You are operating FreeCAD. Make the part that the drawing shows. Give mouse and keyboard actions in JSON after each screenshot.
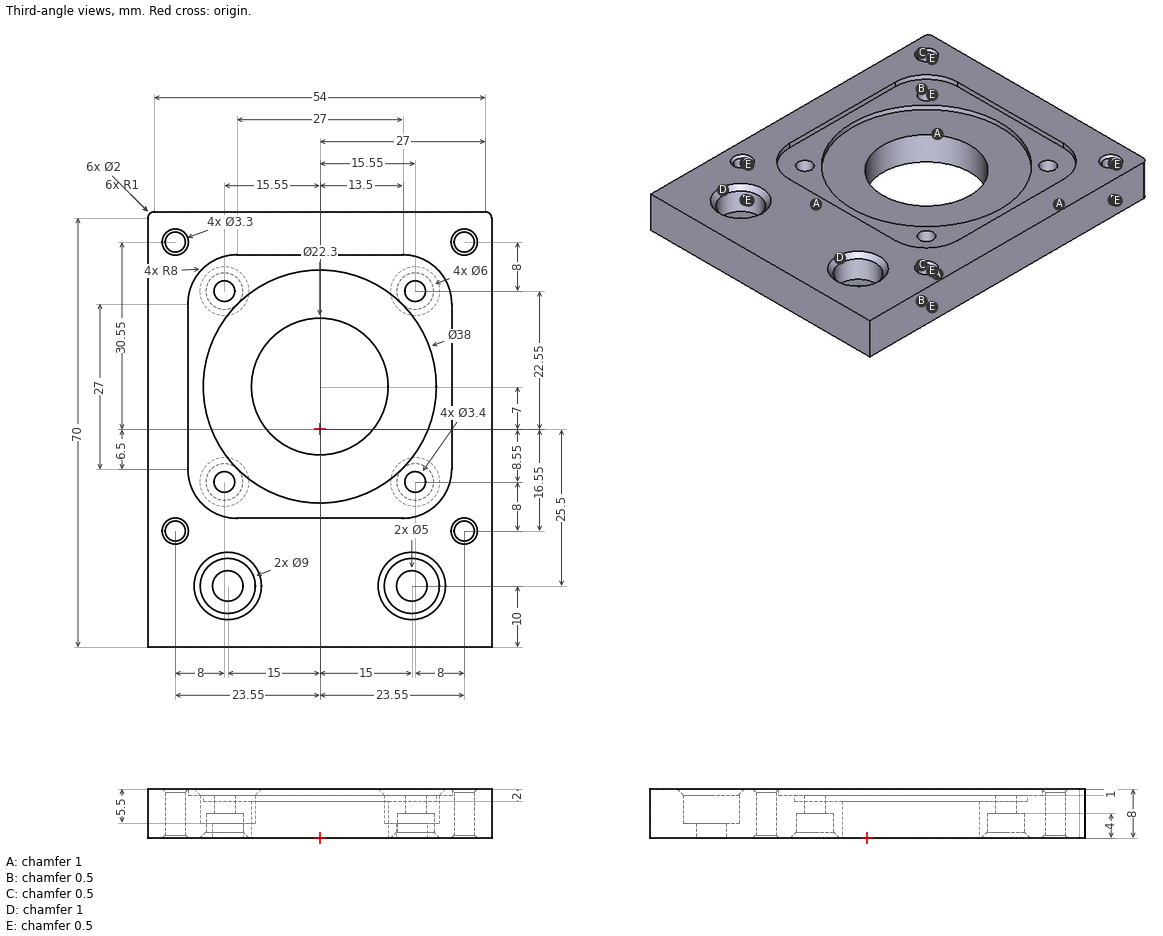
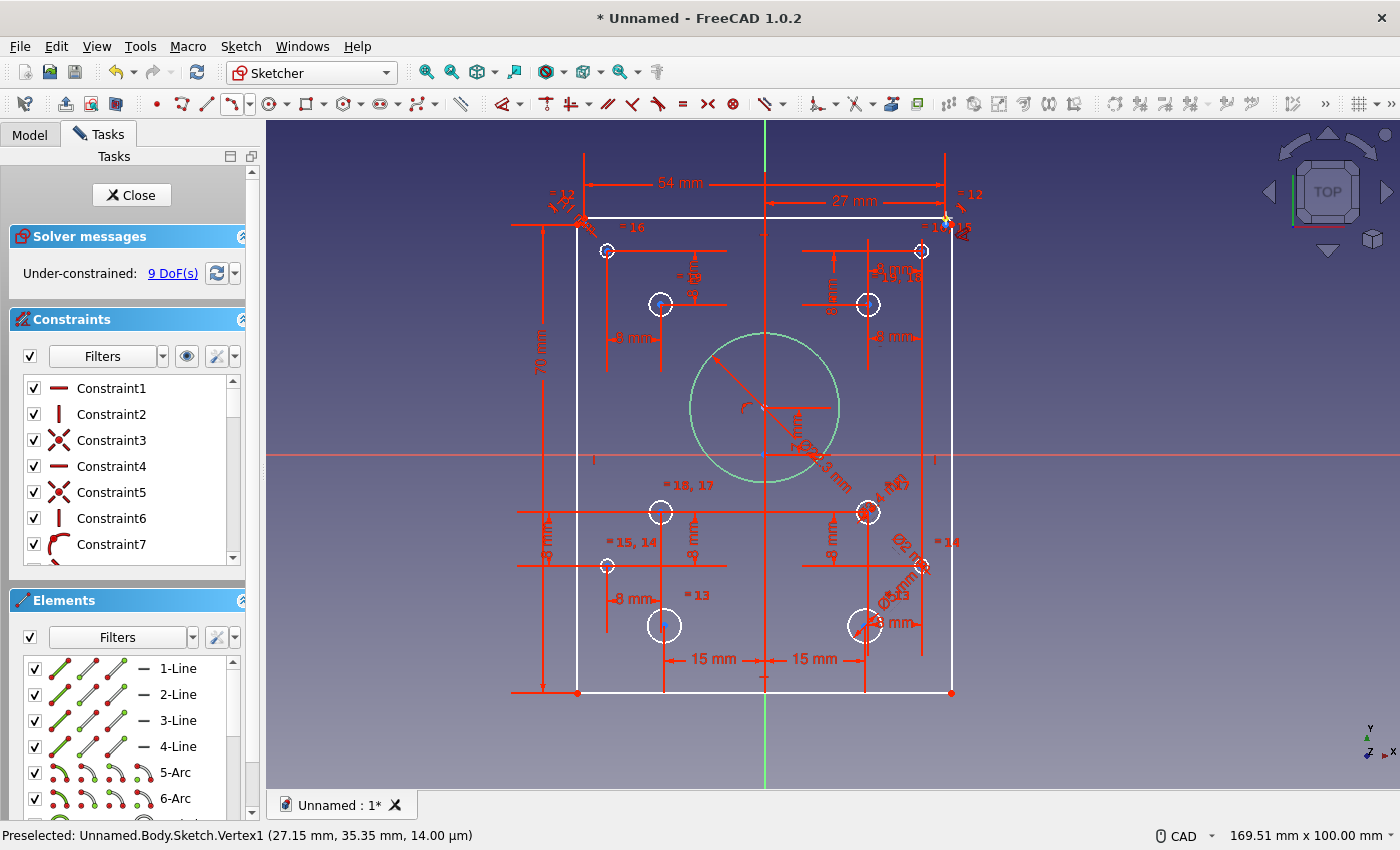
{"action": "left_click", "coordinate": [952, 693]}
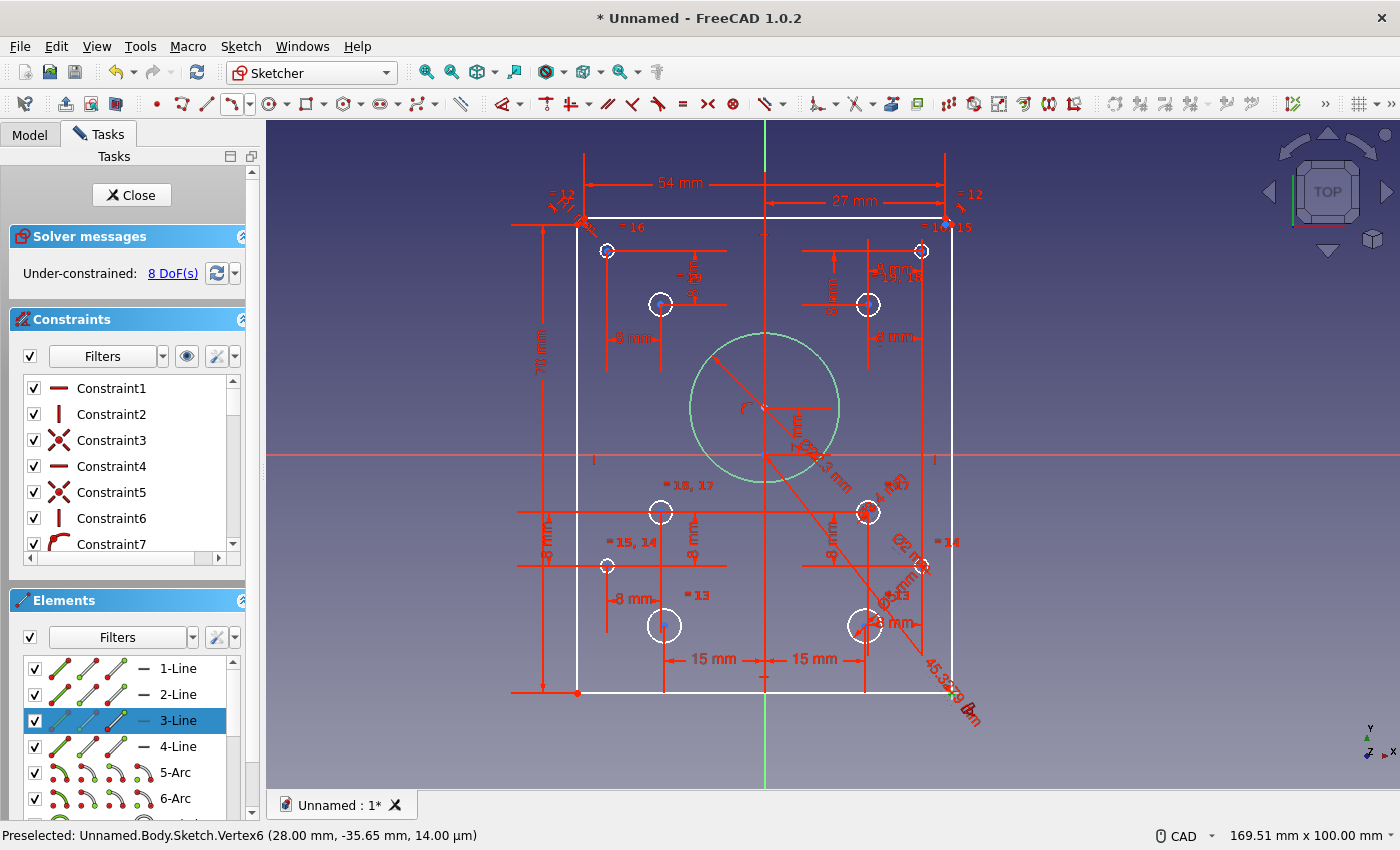
{"action": "left_click", "coordinate": [865, 626]}
{"action": "left_click", "coordinate": [986, 660]}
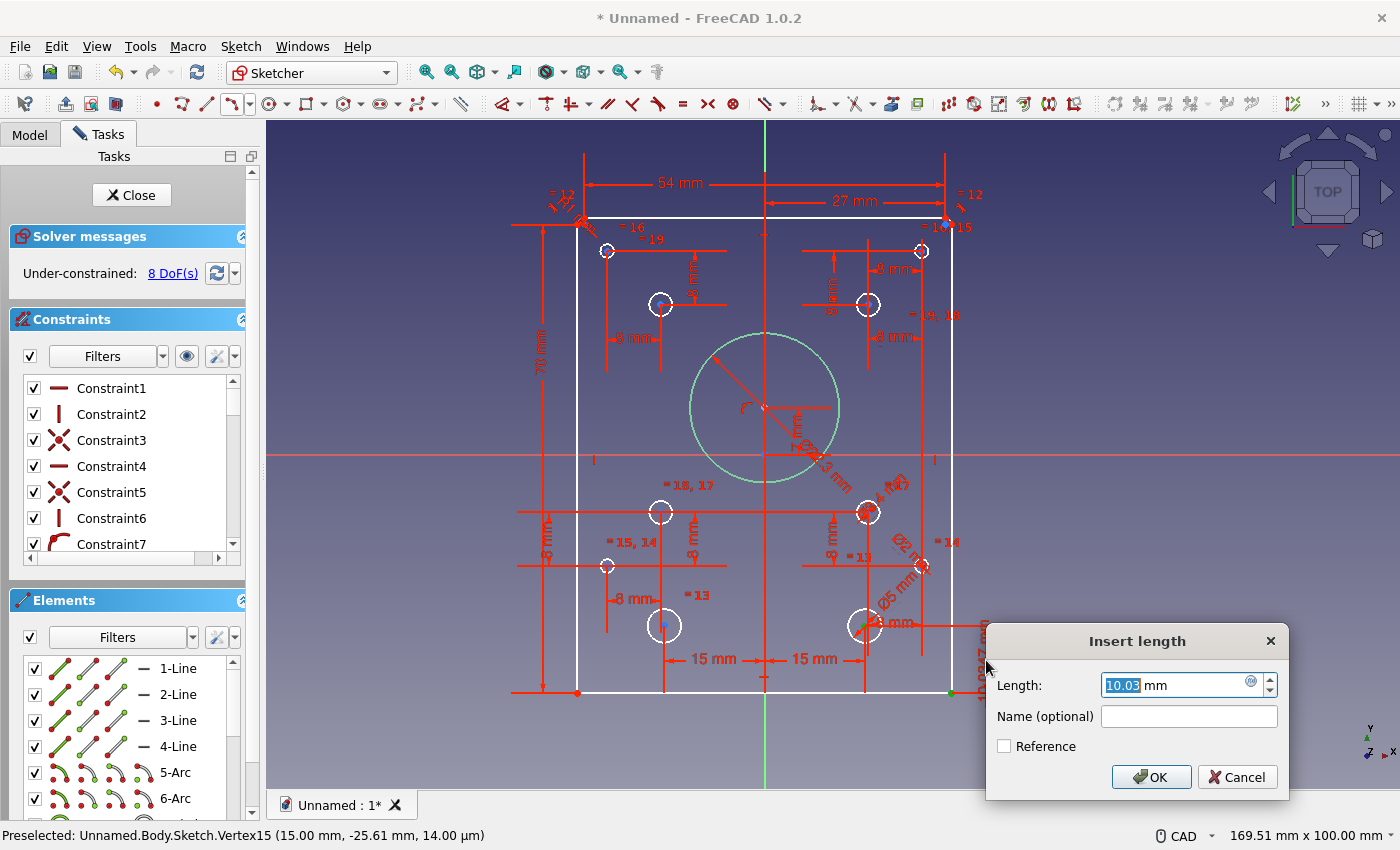
{"action": "type", "text": "10"}
{"action": "key", "text": "Return"}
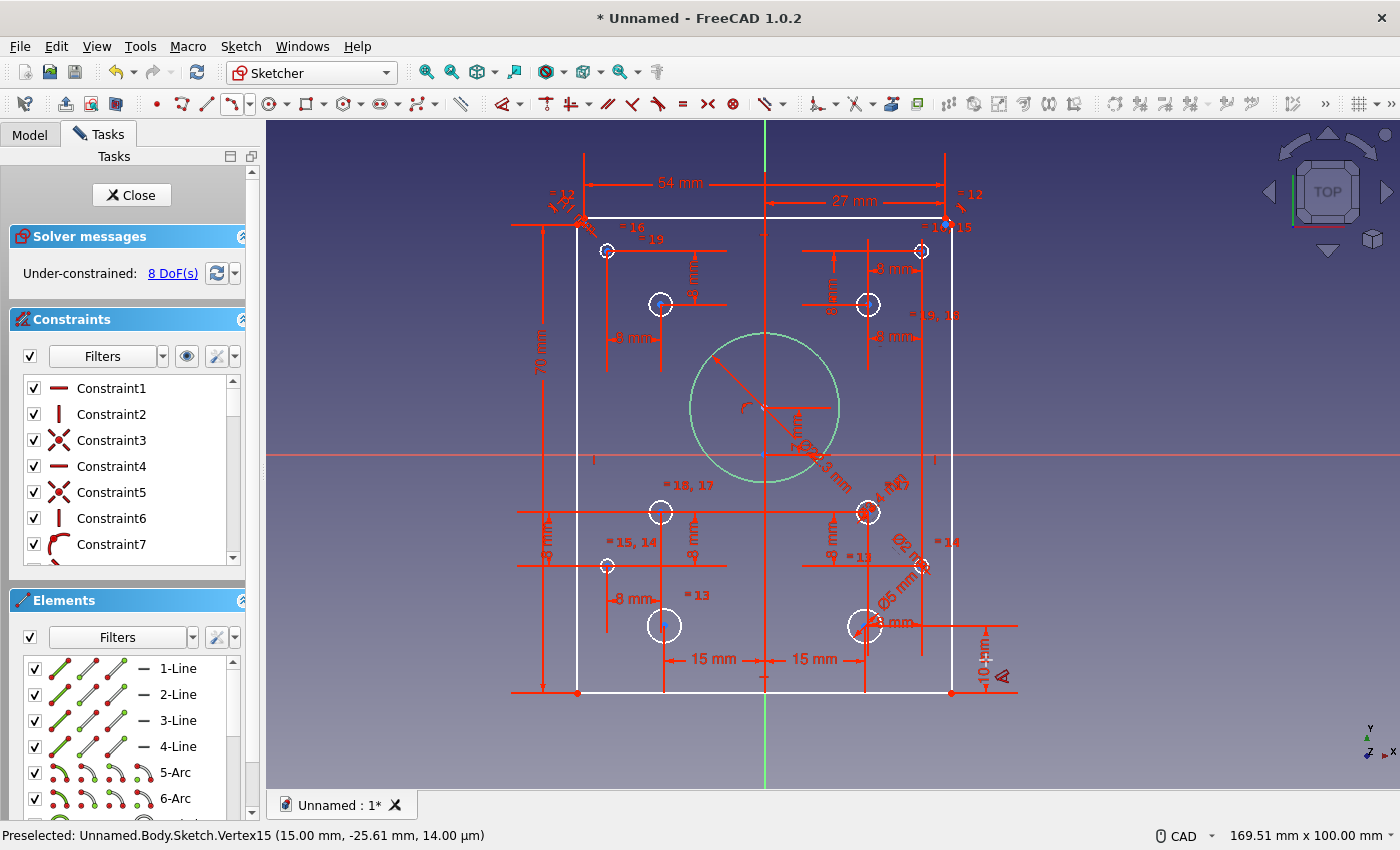
{"action": "left_click", "coordinate": [577, 693]}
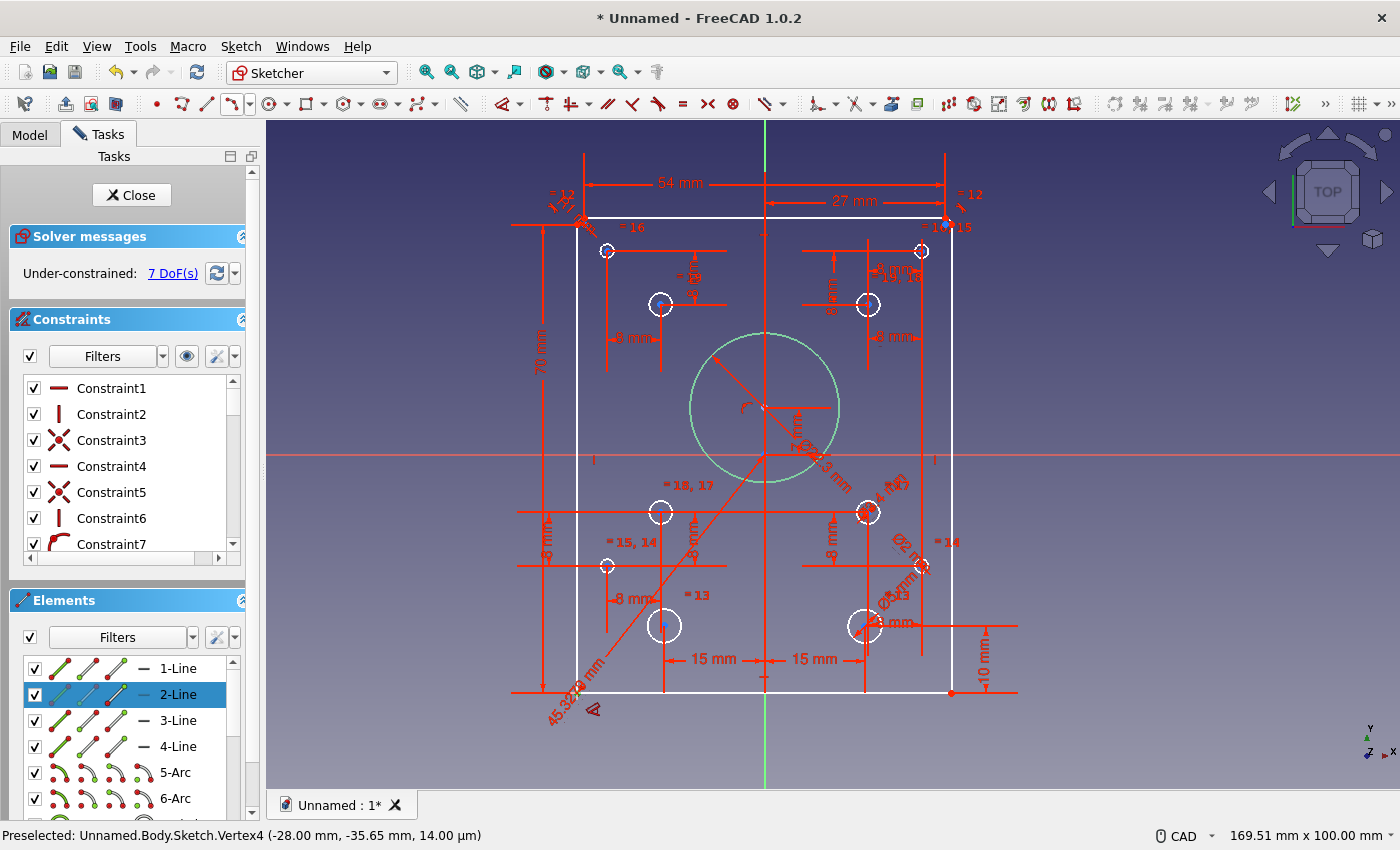
{"action": "left_click", "coordinate": [664, 626]}
{"action": "left_click", "coordinate": [543, 660]}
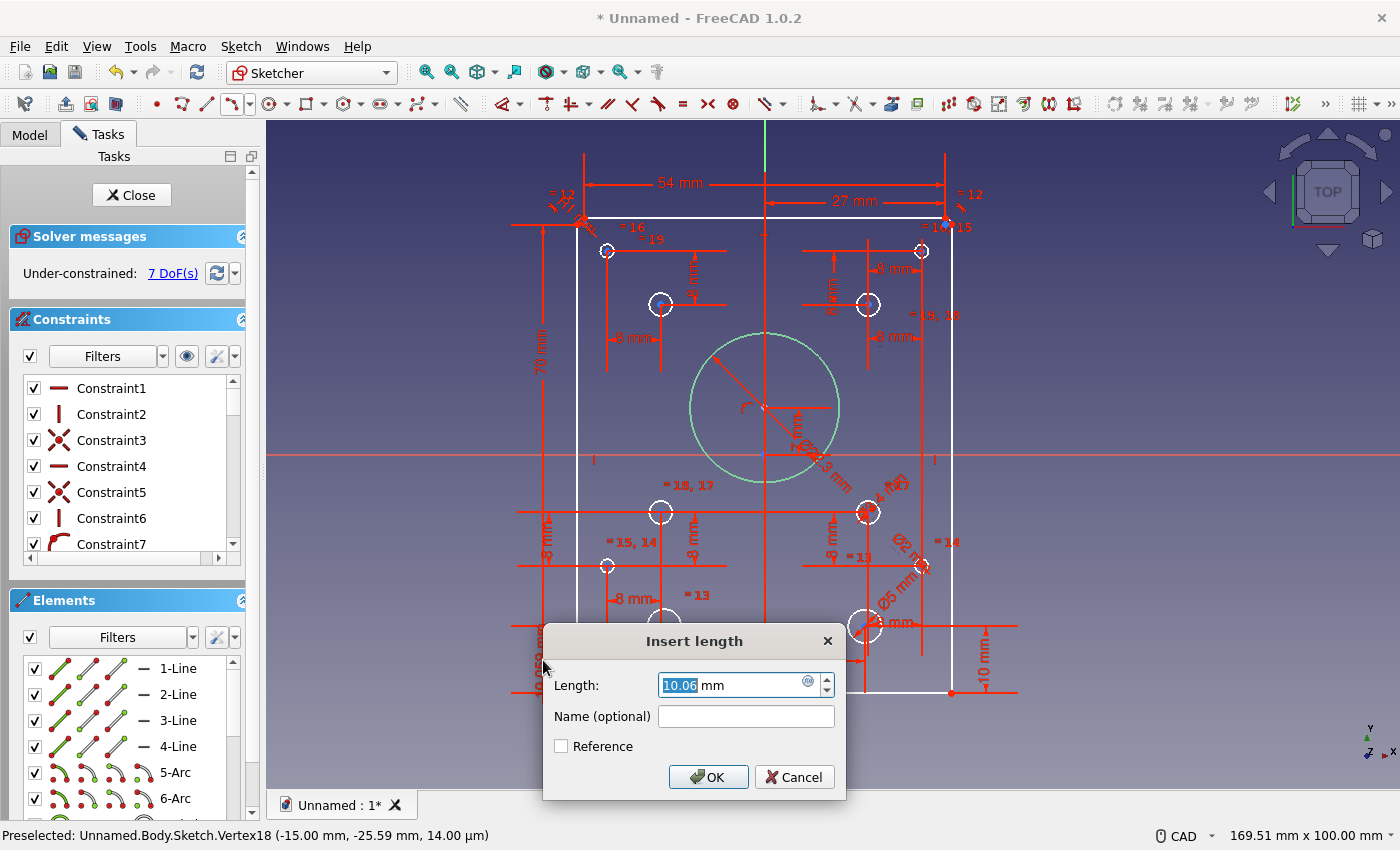
{"action": "type", "text": "10"}
{"action": "key", "text": "Return"}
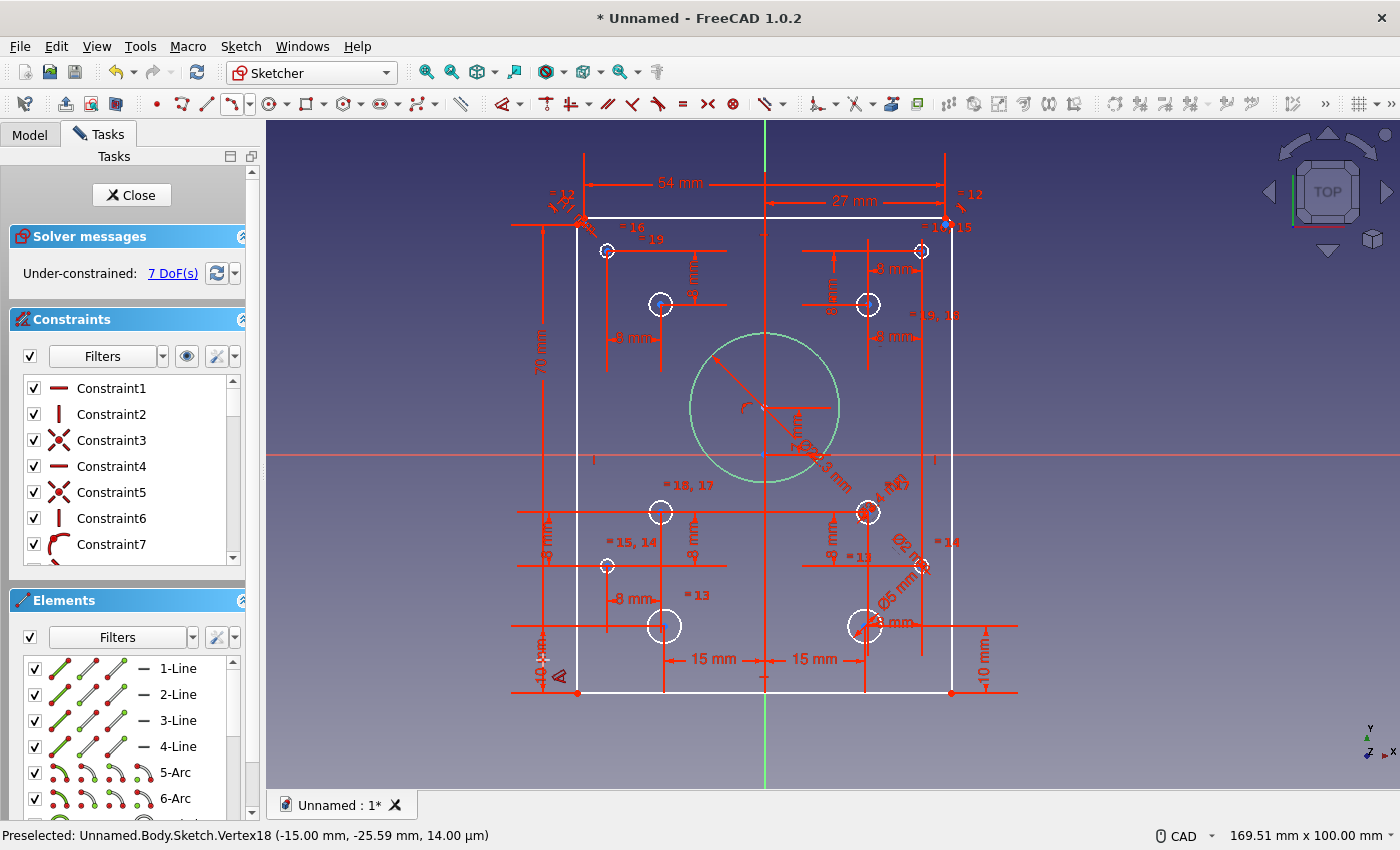
{"action": "left_click", "coordinate": [865, 626]}
{"action": "left_click", "coordinate": [731, 501]}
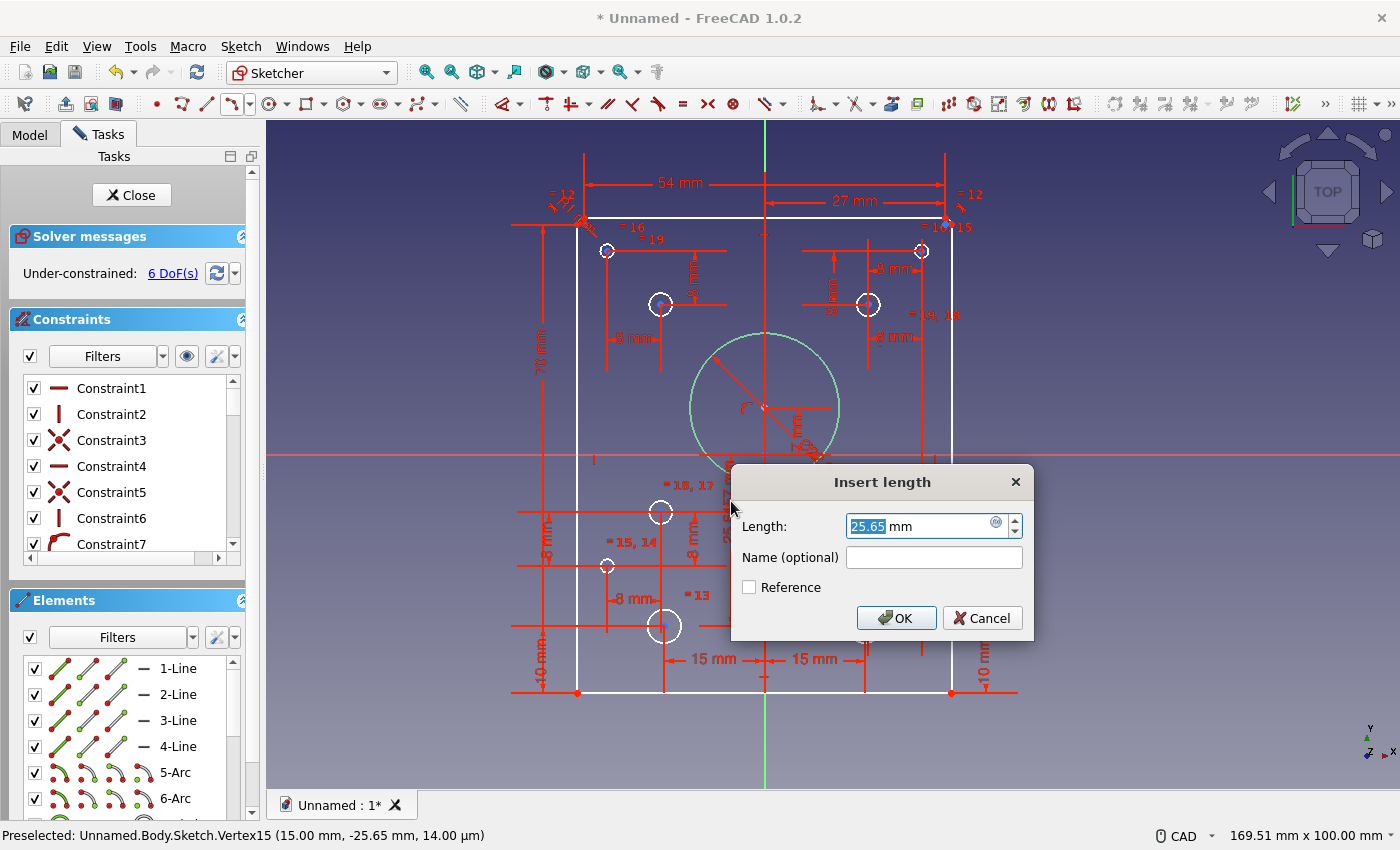
{"action": "type", "text": "25.5"}
{"action": "key", "text": "Return"}